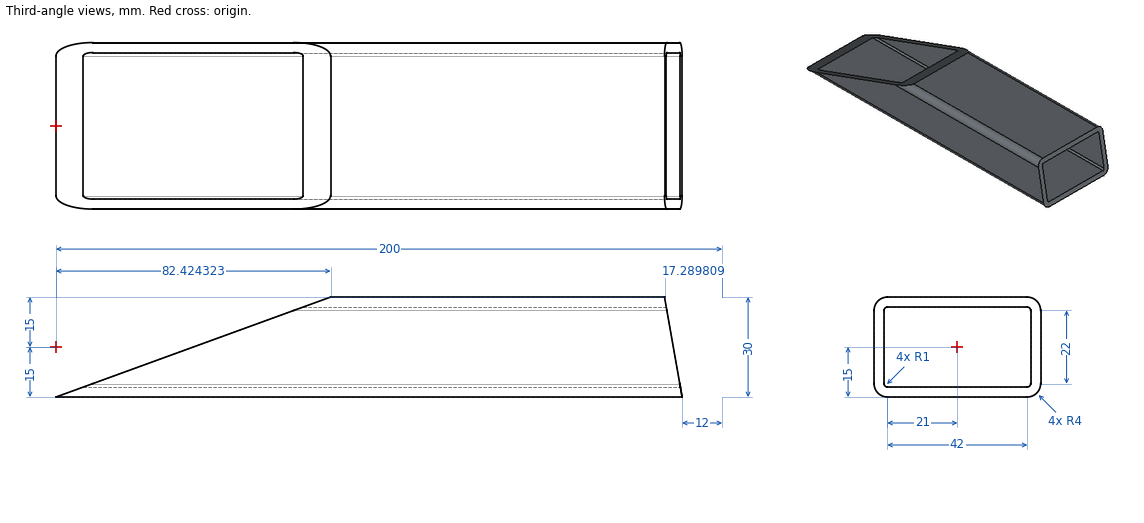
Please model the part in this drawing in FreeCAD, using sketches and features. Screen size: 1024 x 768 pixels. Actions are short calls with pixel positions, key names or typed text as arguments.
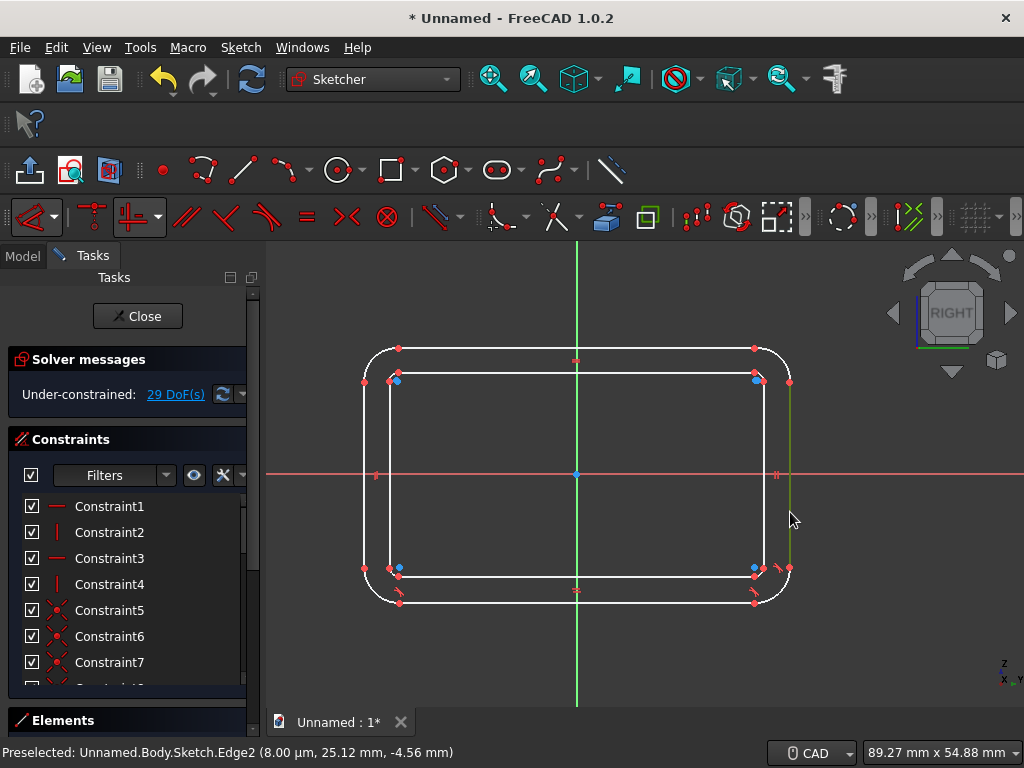
click(786, 366)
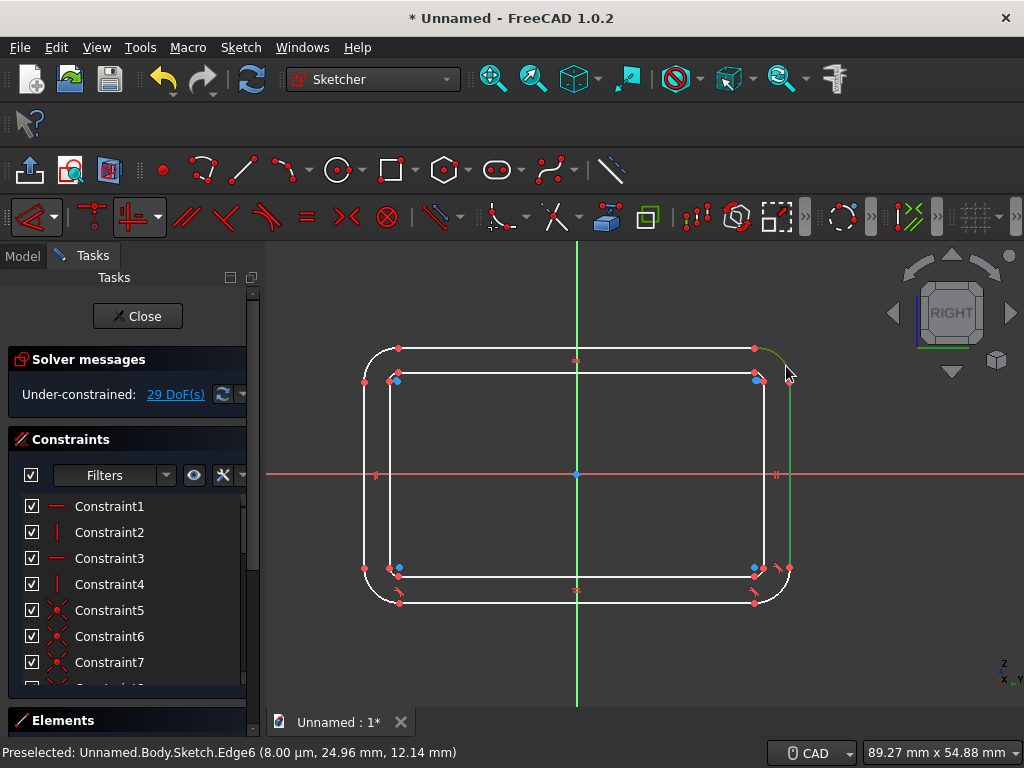
click(268, 218)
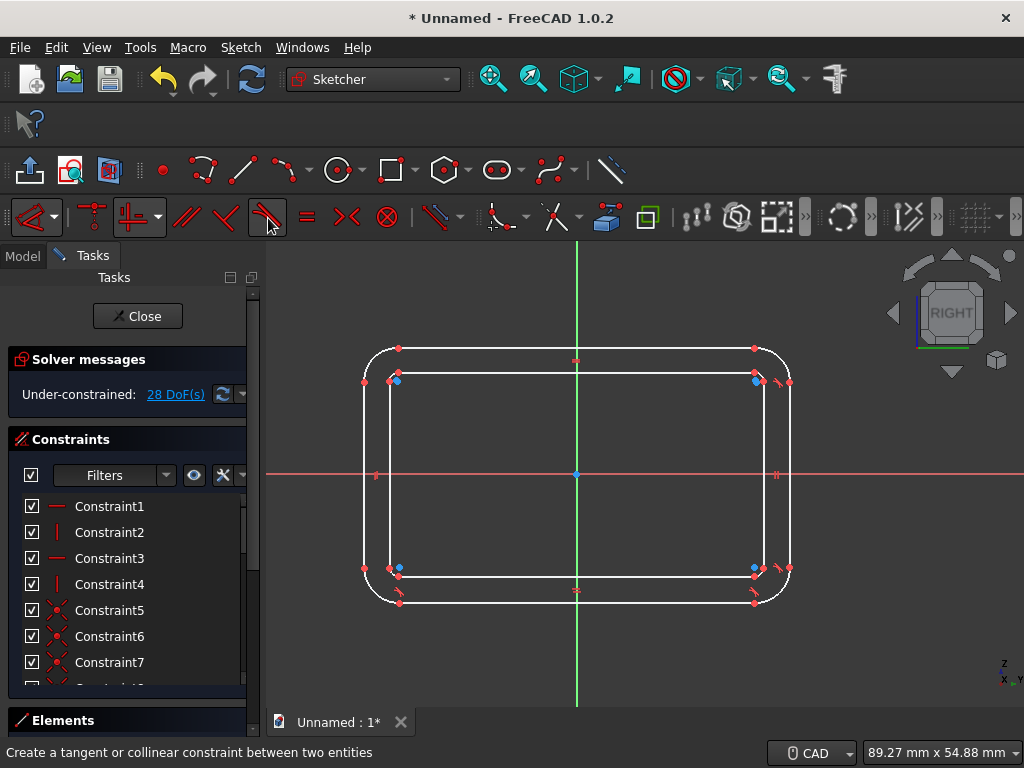
click(648, 348)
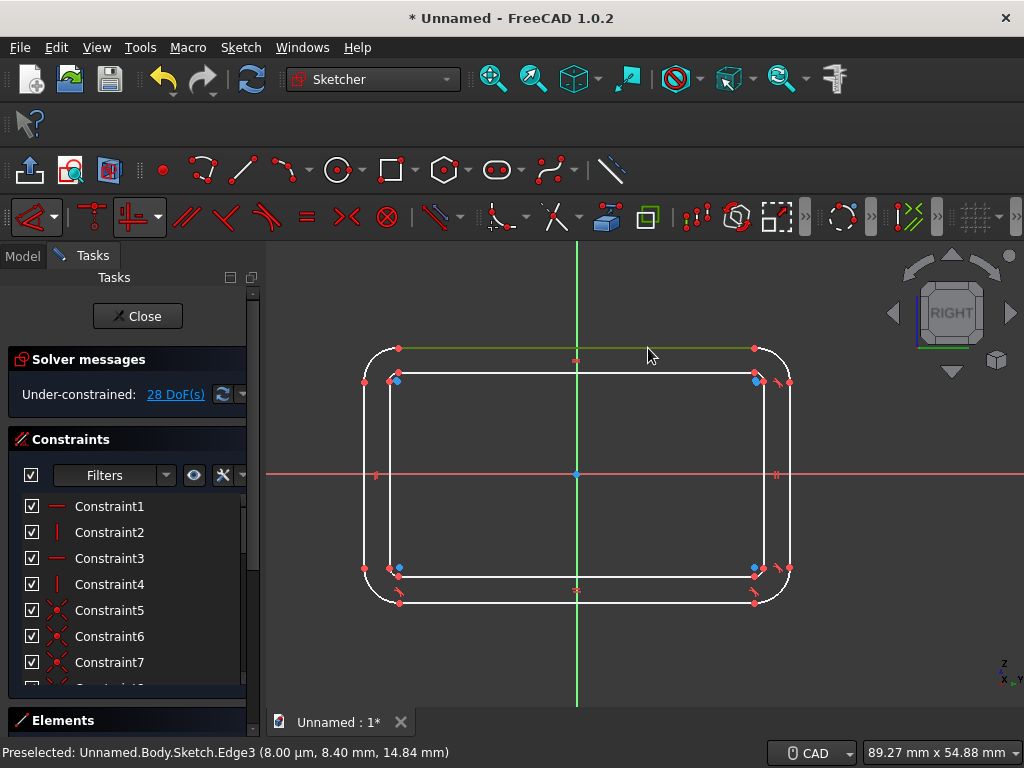
click(786, 366)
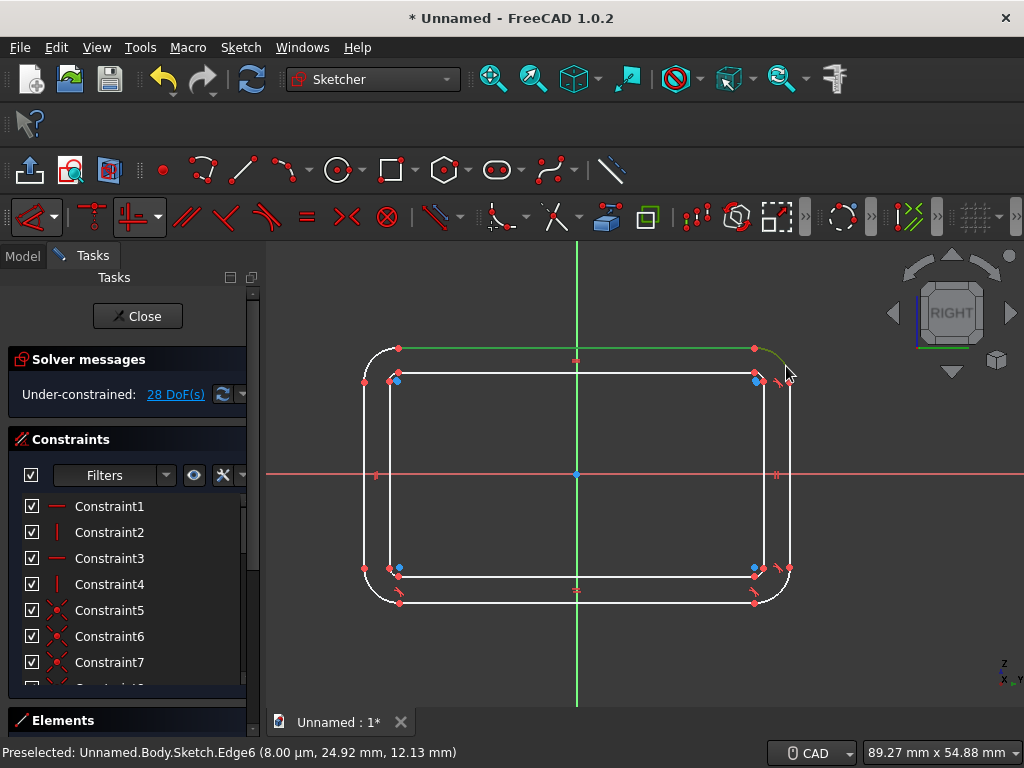
click(268, 218)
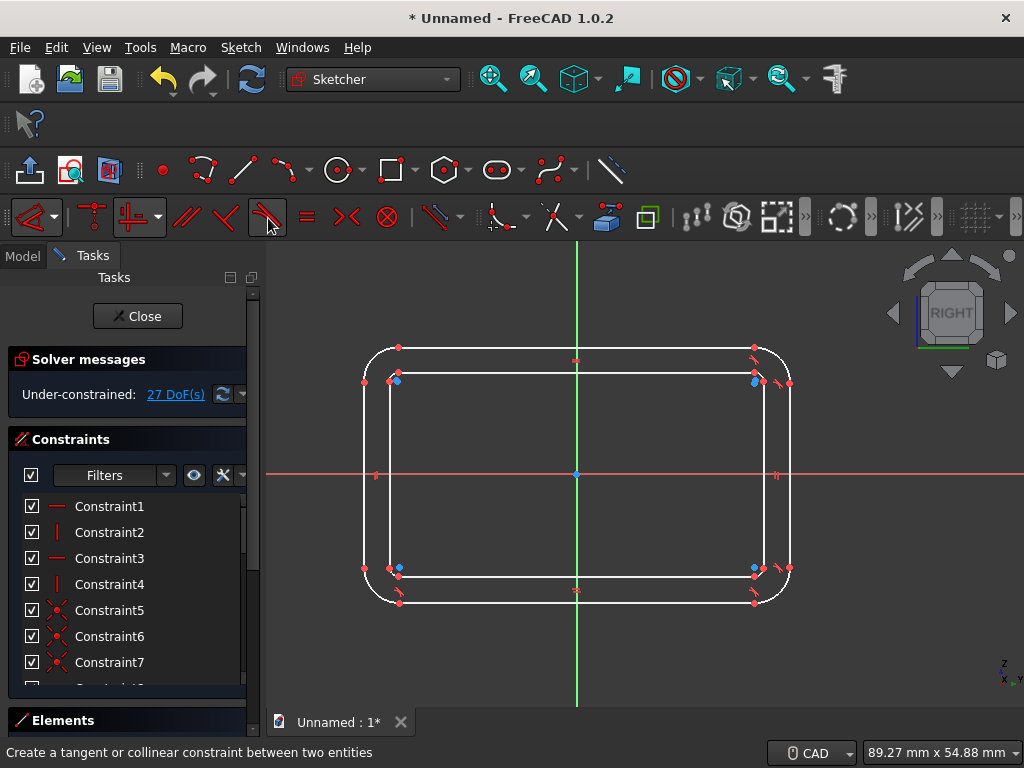
click(648, 348)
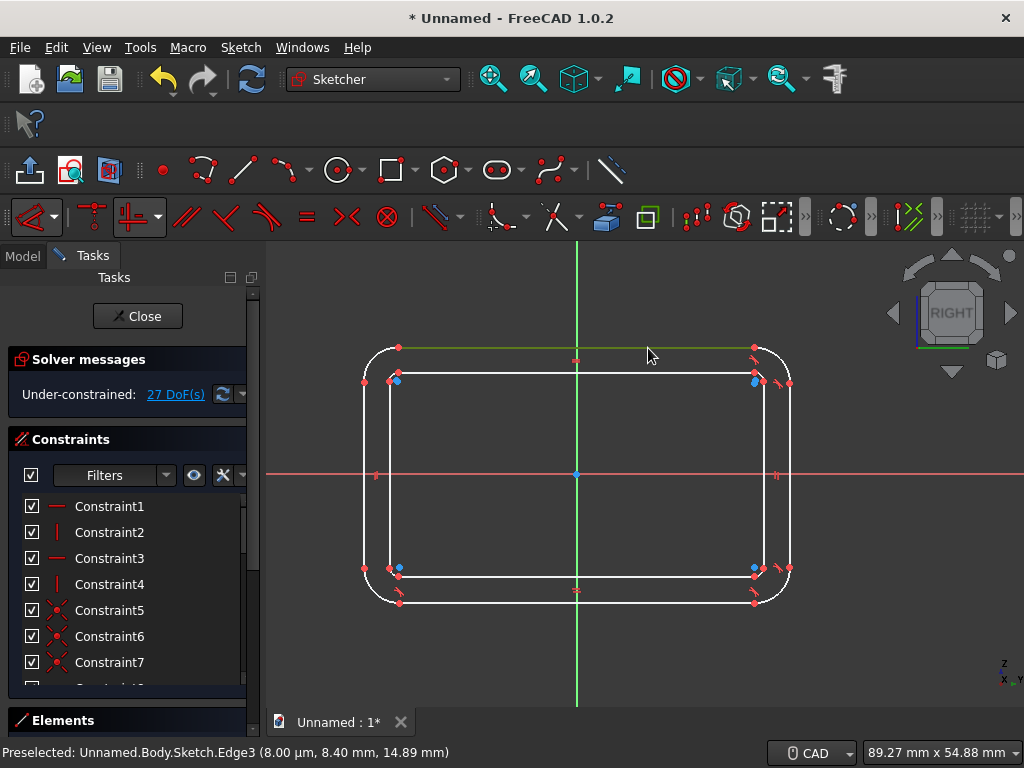
click(382, 351)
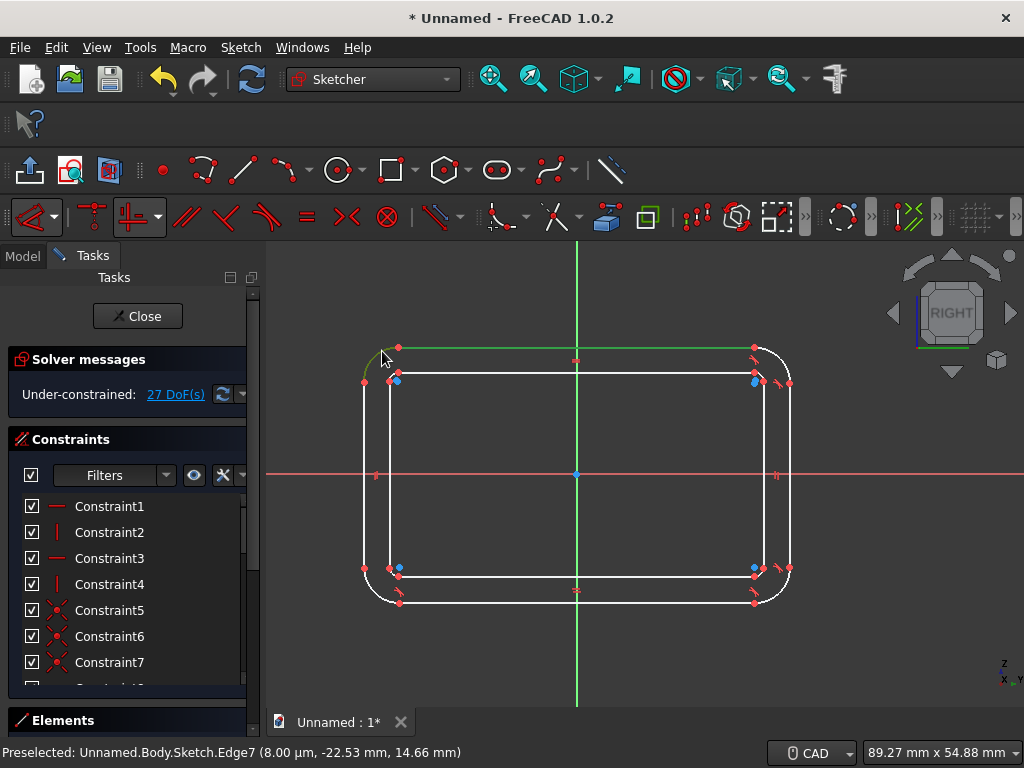
click(268, 218)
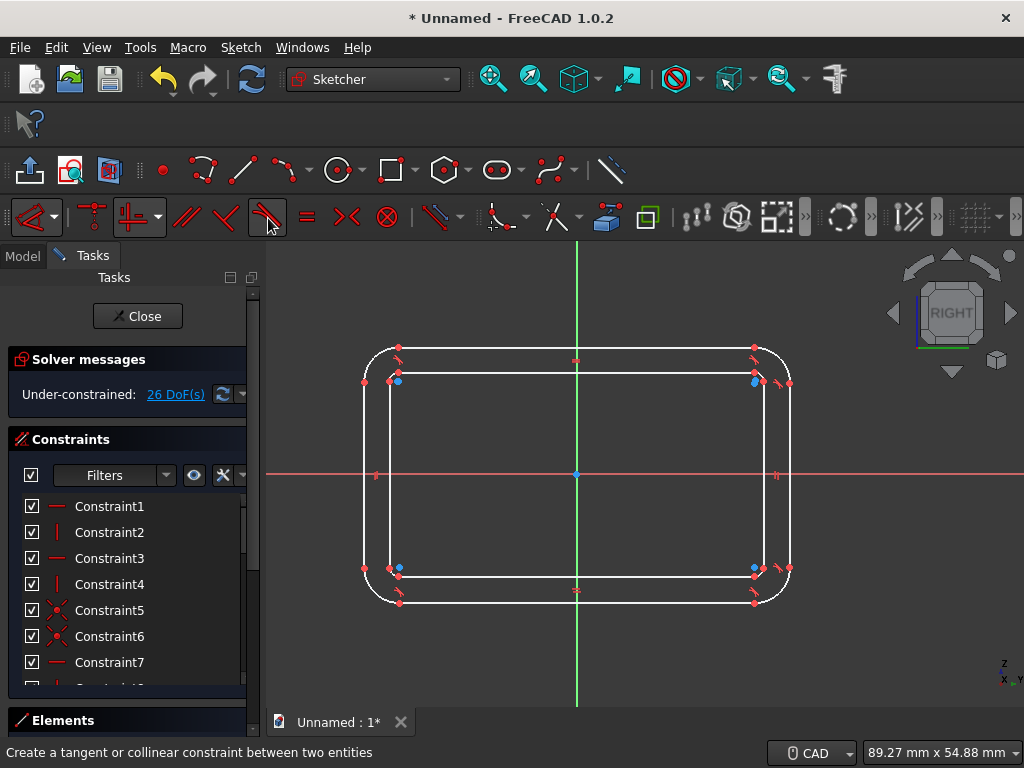
click(364, 438)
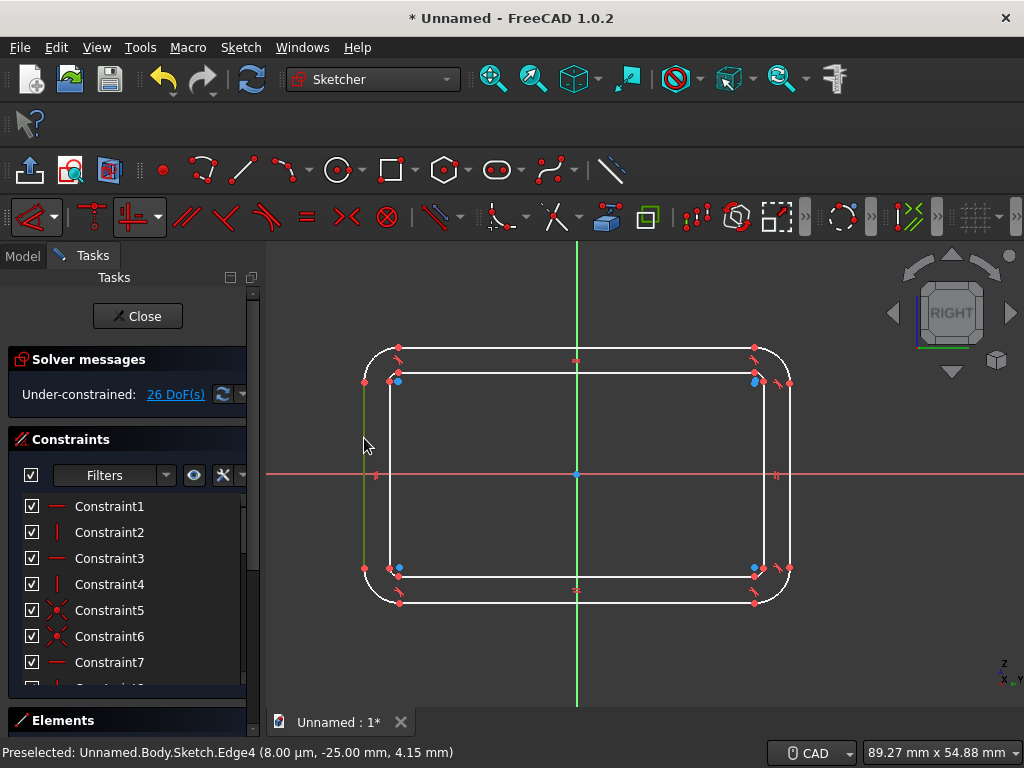
click(383, 352)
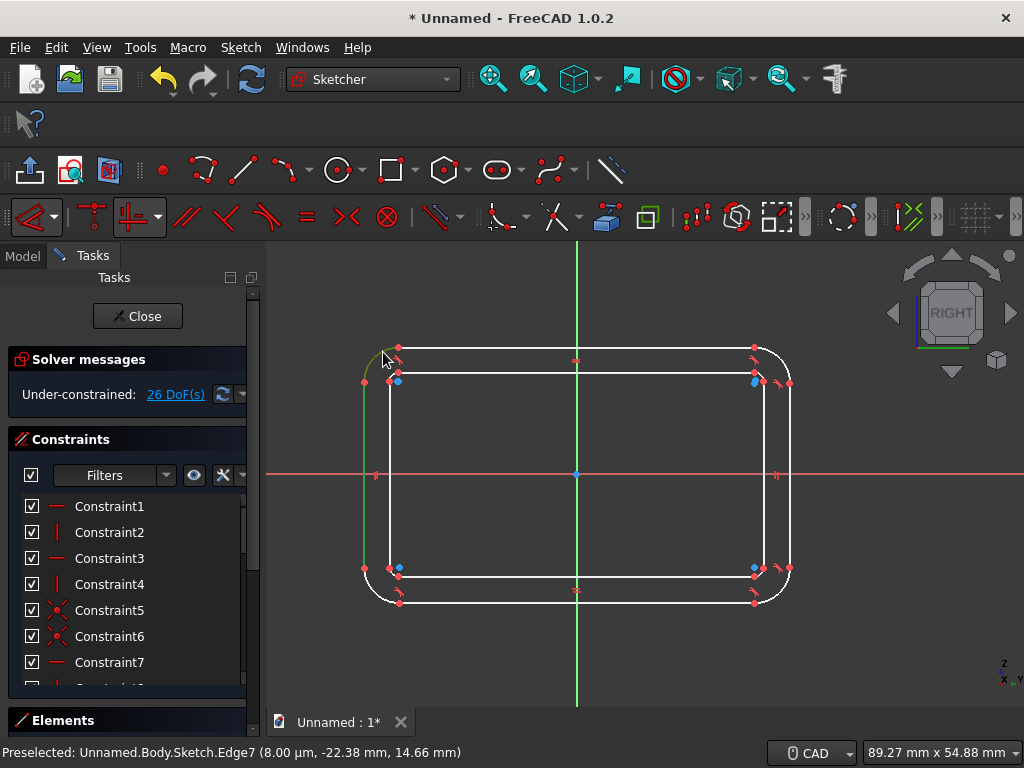
click(268, 218)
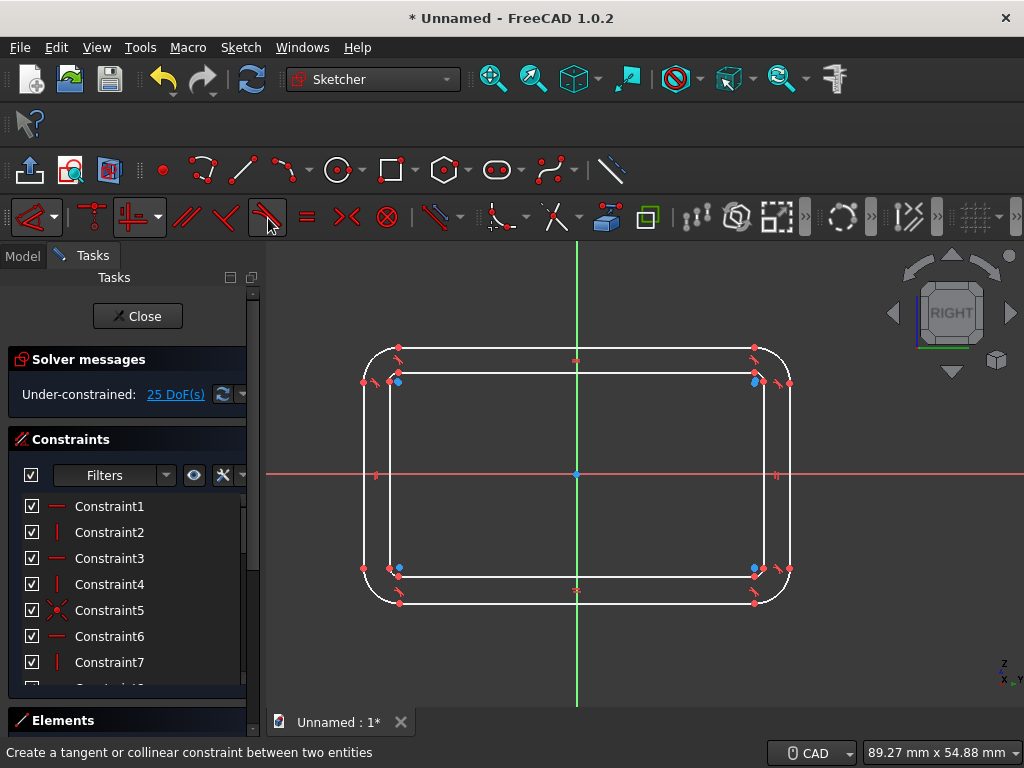
click(364, 438)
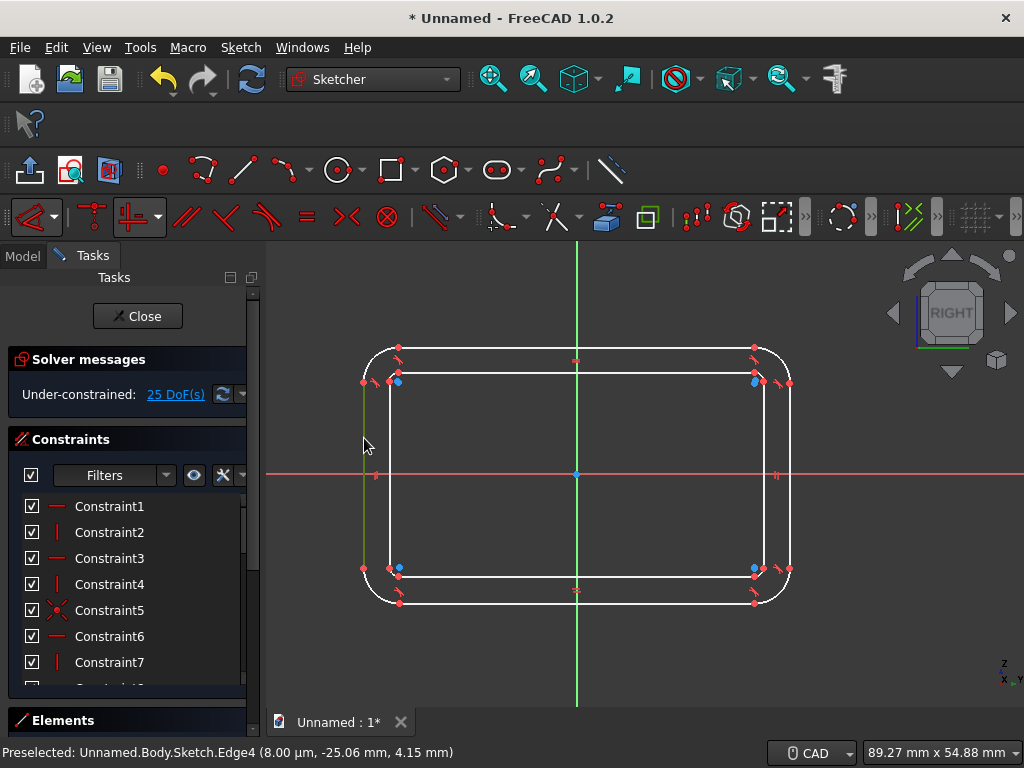
click(368, 584)